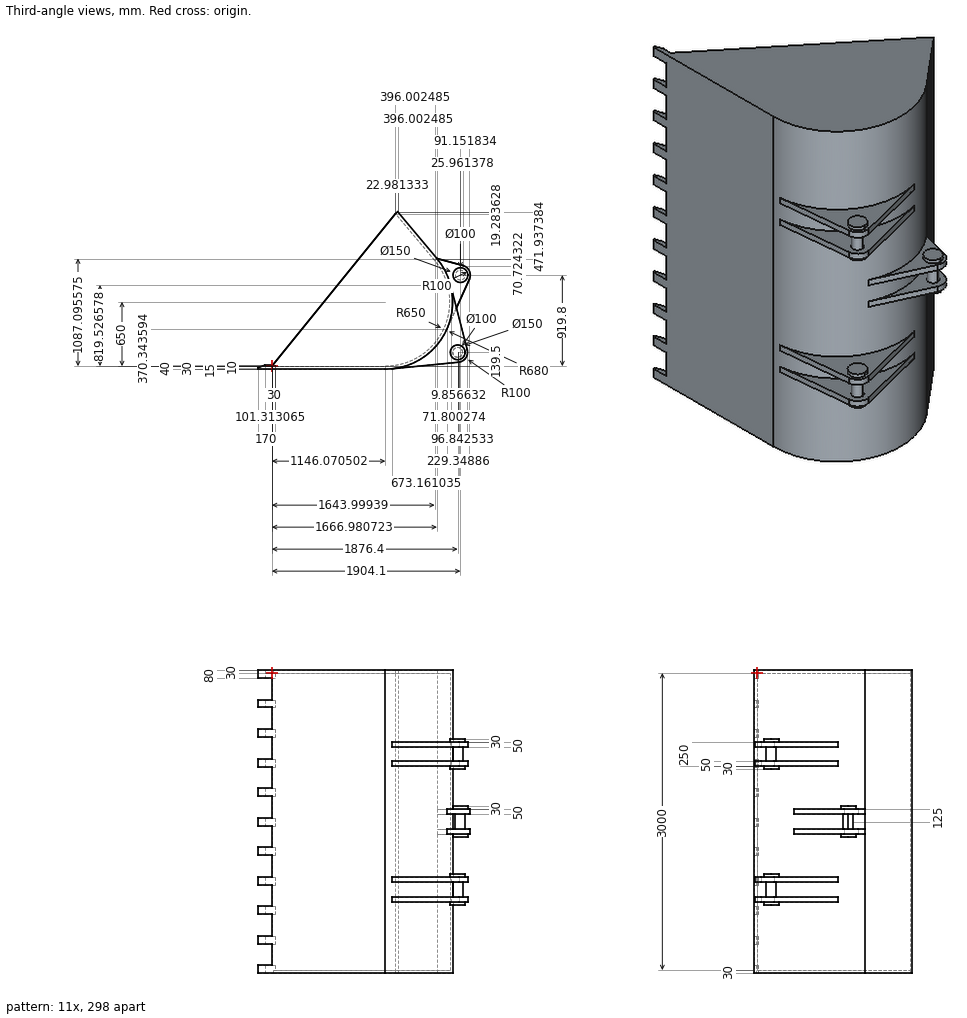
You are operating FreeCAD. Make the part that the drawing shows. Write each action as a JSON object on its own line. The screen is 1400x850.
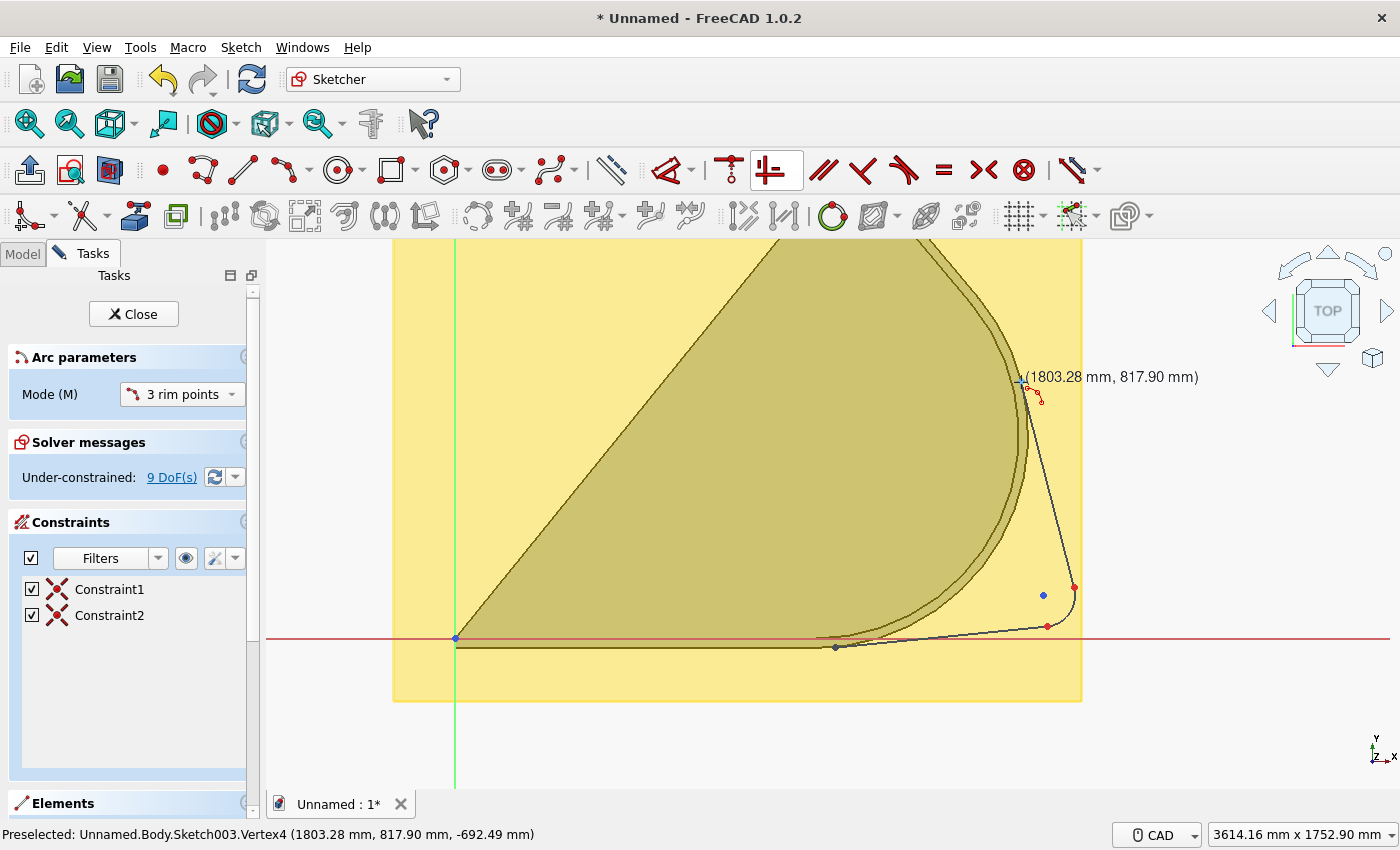
{"action": "scroll", "coordinate": [836, 647], "scroll_direction": "up", "scroll_amount": 4}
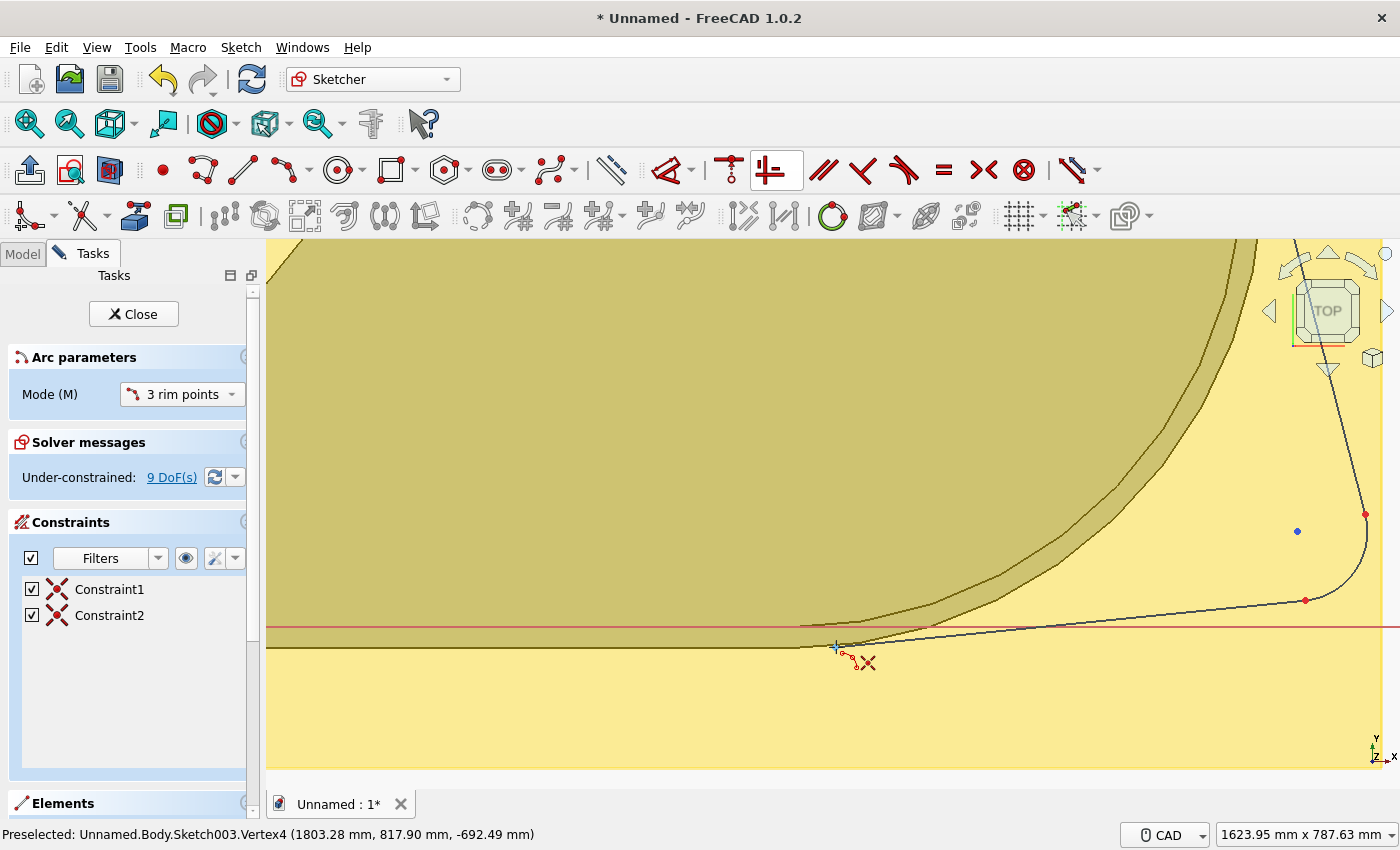
{"action": "left_click", "coordinate": [835, 647]}
{"action": "left_click", "coordinate": [1177, 446]}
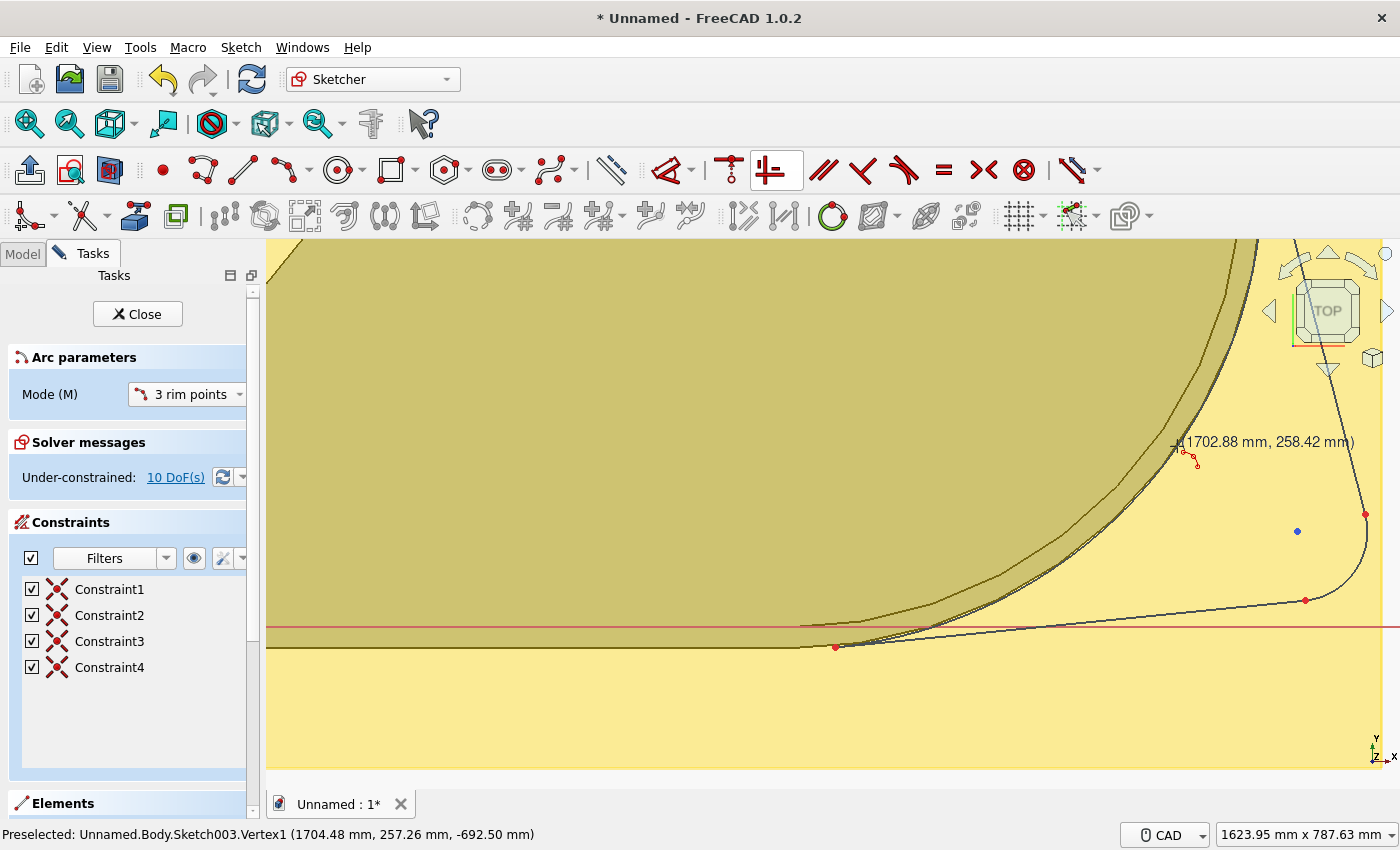
{"action": "left_click", "coordinate": [338, 170]}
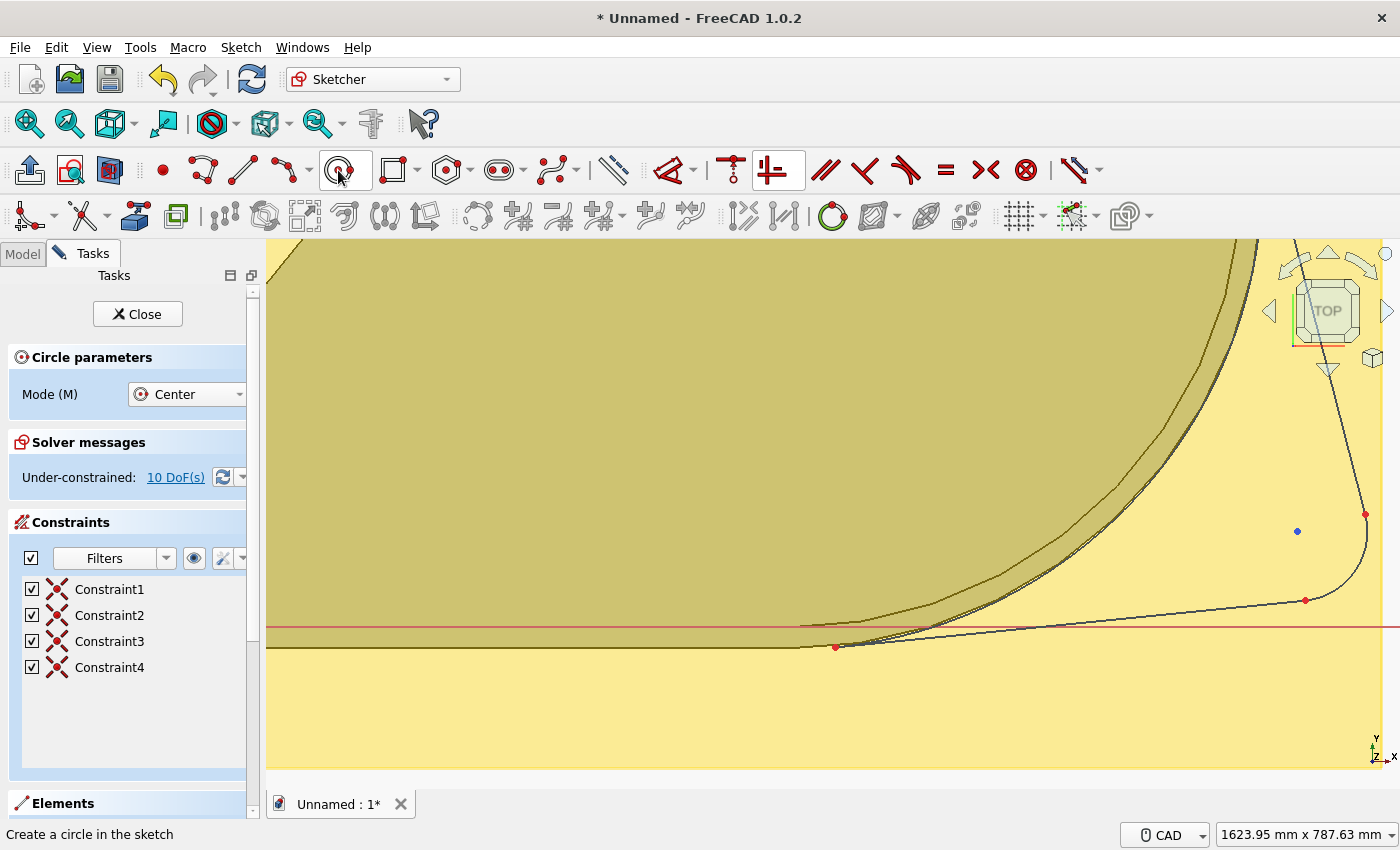
{"action": "scroll", "coordinate": [836, 647], "scroll_direction": "down", "scroll_amount": 4}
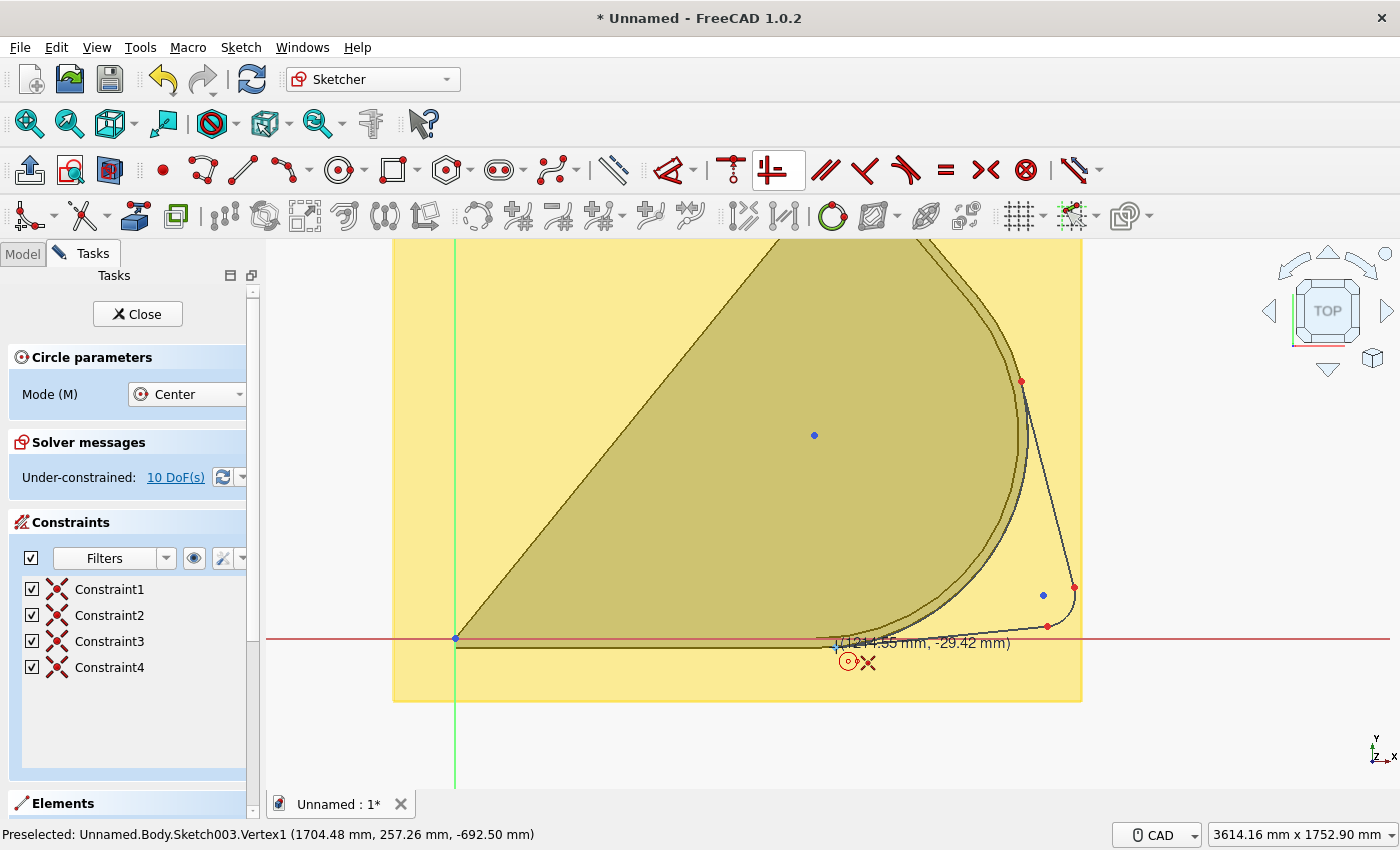
{"action": "scroll", "coordinate": [1044, 595], "scroll_direction": "up", "scroll_amount": 2}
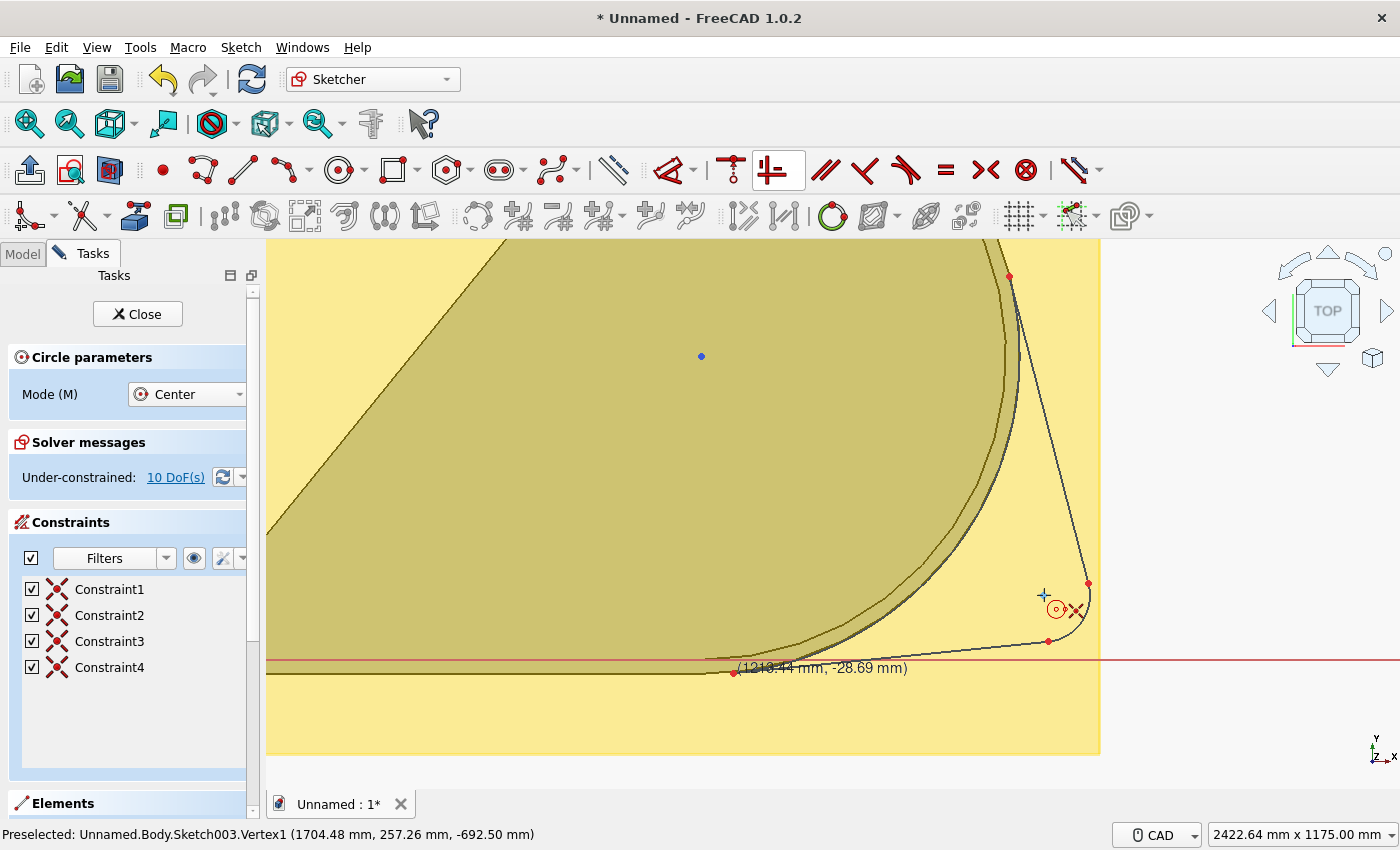
{"action": "left_click", "coordinate": [1044, 594]}
{"action": "left_click", "coordinate": [1060, 578]}
{"action": "key", "text": "Escape"}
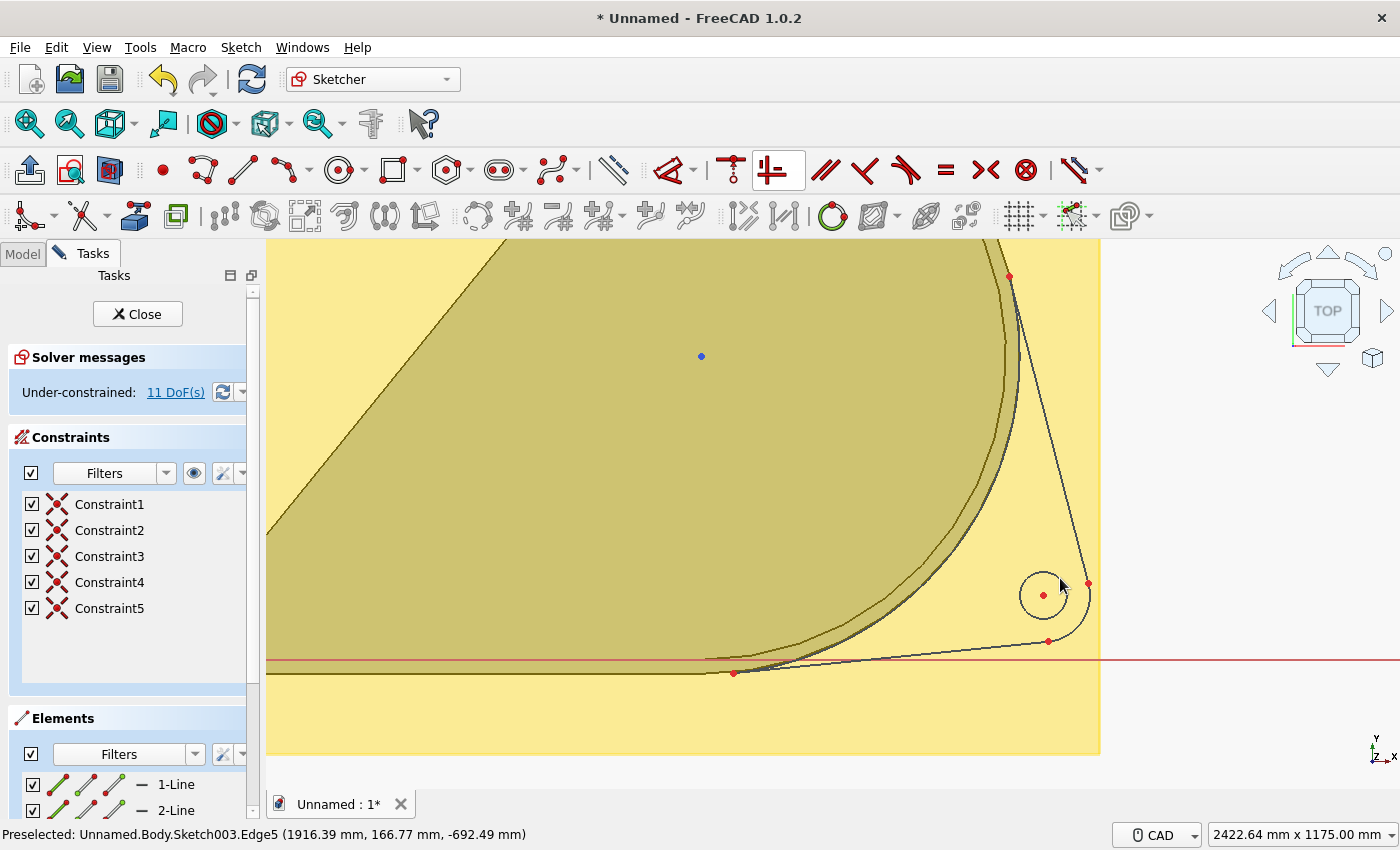
{"action": "key", "text": "d"}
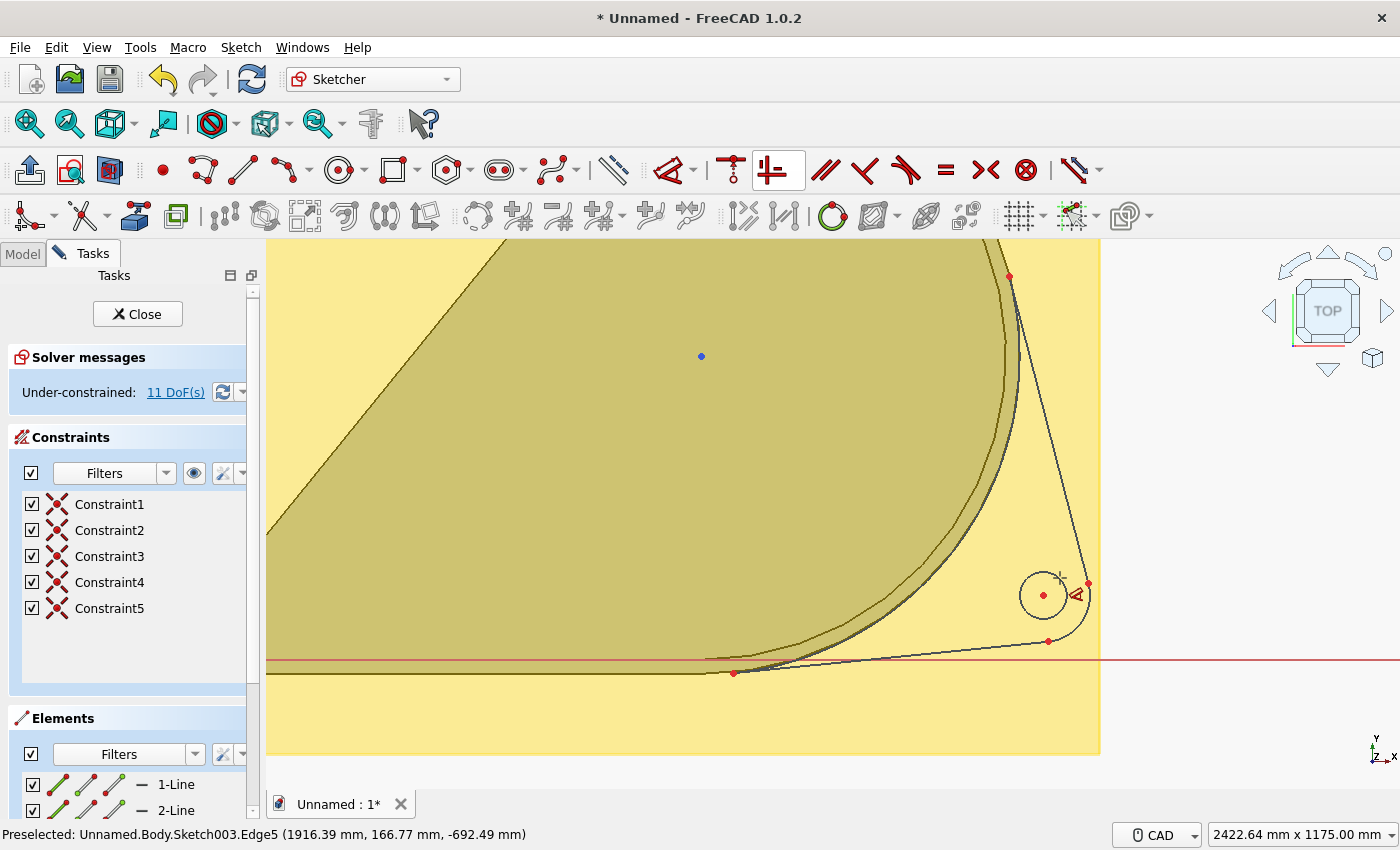
{"action": "left_click", "coordinate": [1071, 633]}
{"action": "left_click", "coordinate": [1054, 673]}